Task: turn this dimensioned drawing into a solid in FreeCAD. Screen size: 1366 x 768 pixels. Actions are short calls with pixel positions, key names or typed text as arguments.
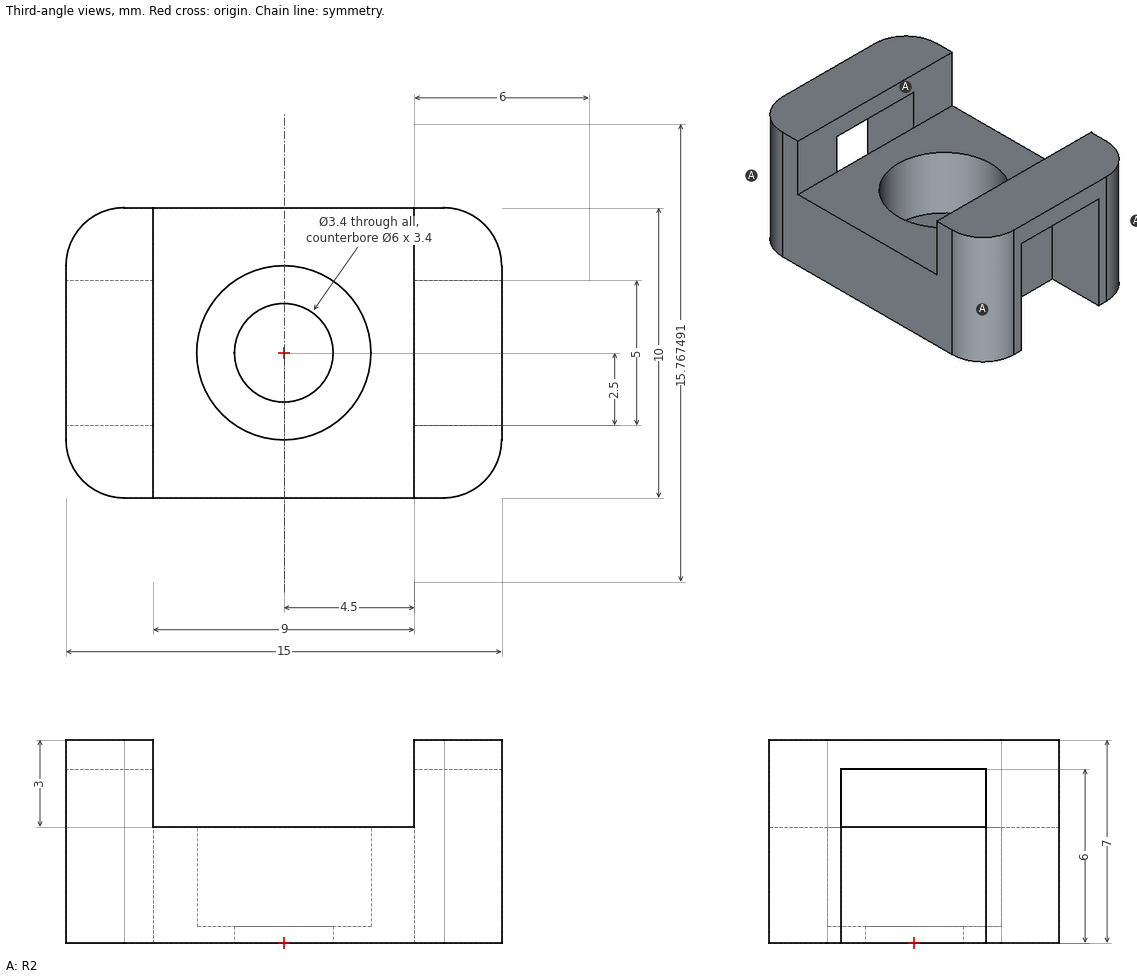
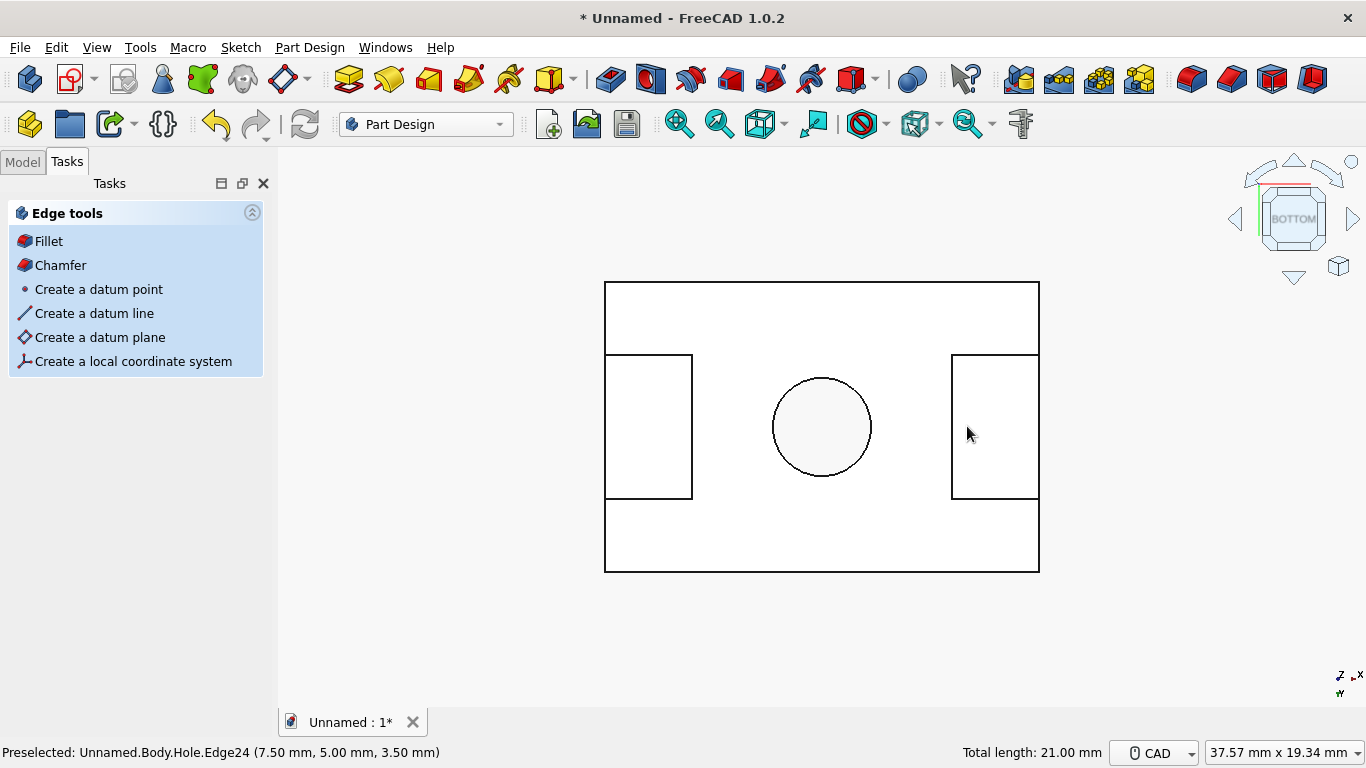
key(4)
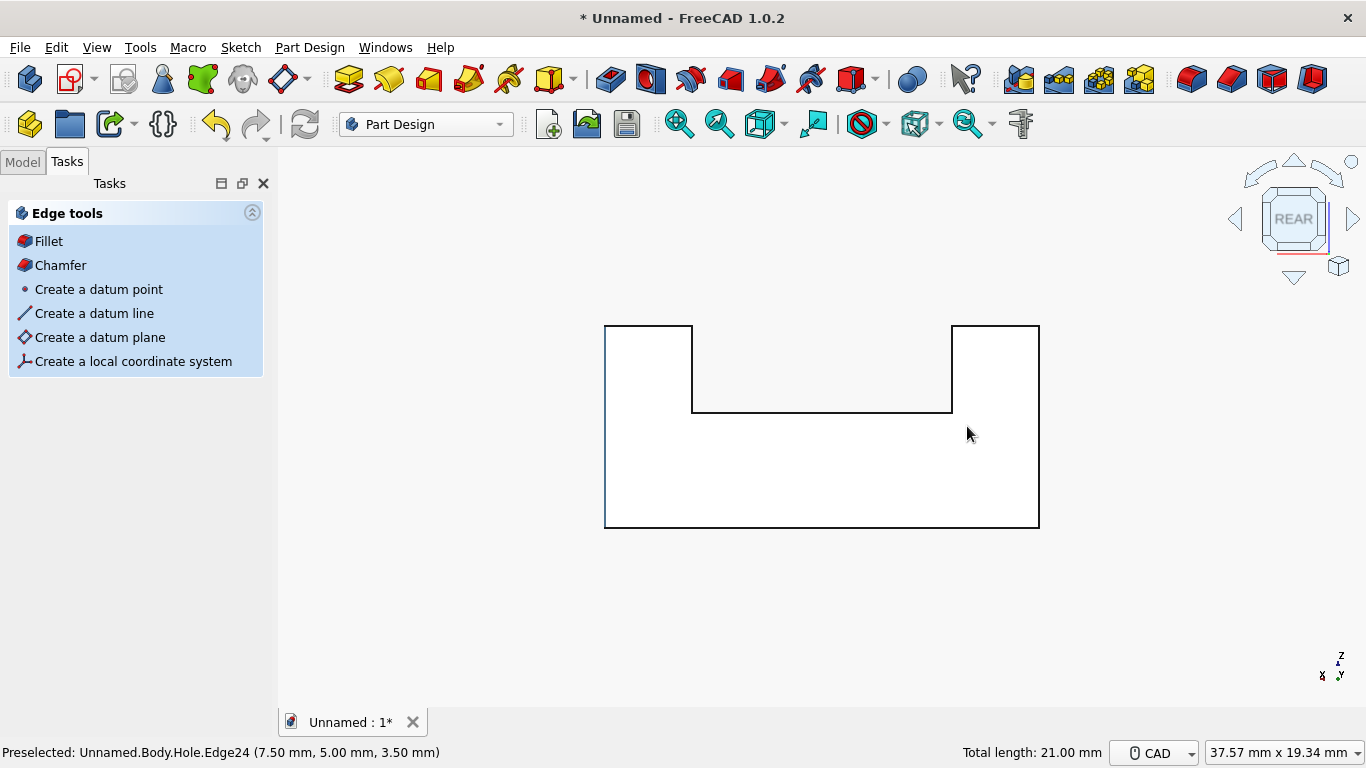
click(680, 124)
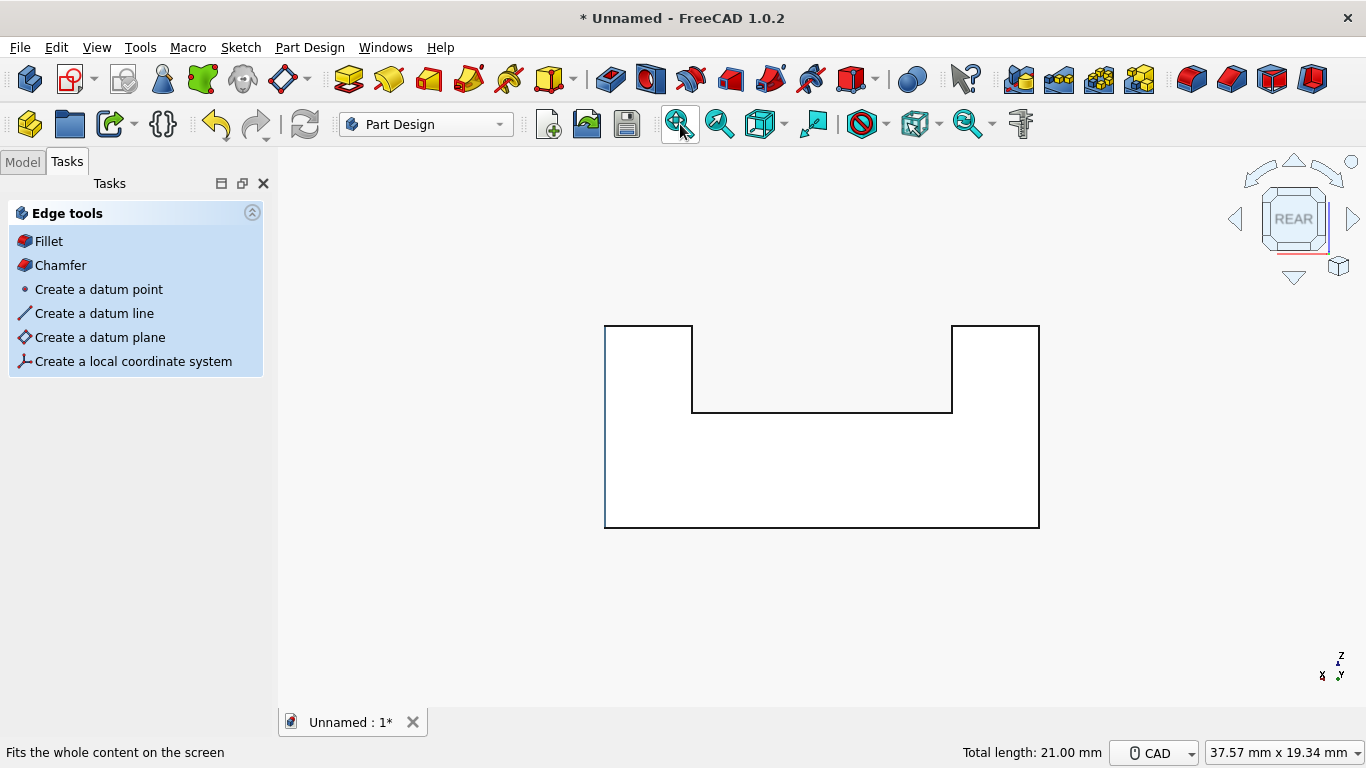
click(1039, 426, ctrl)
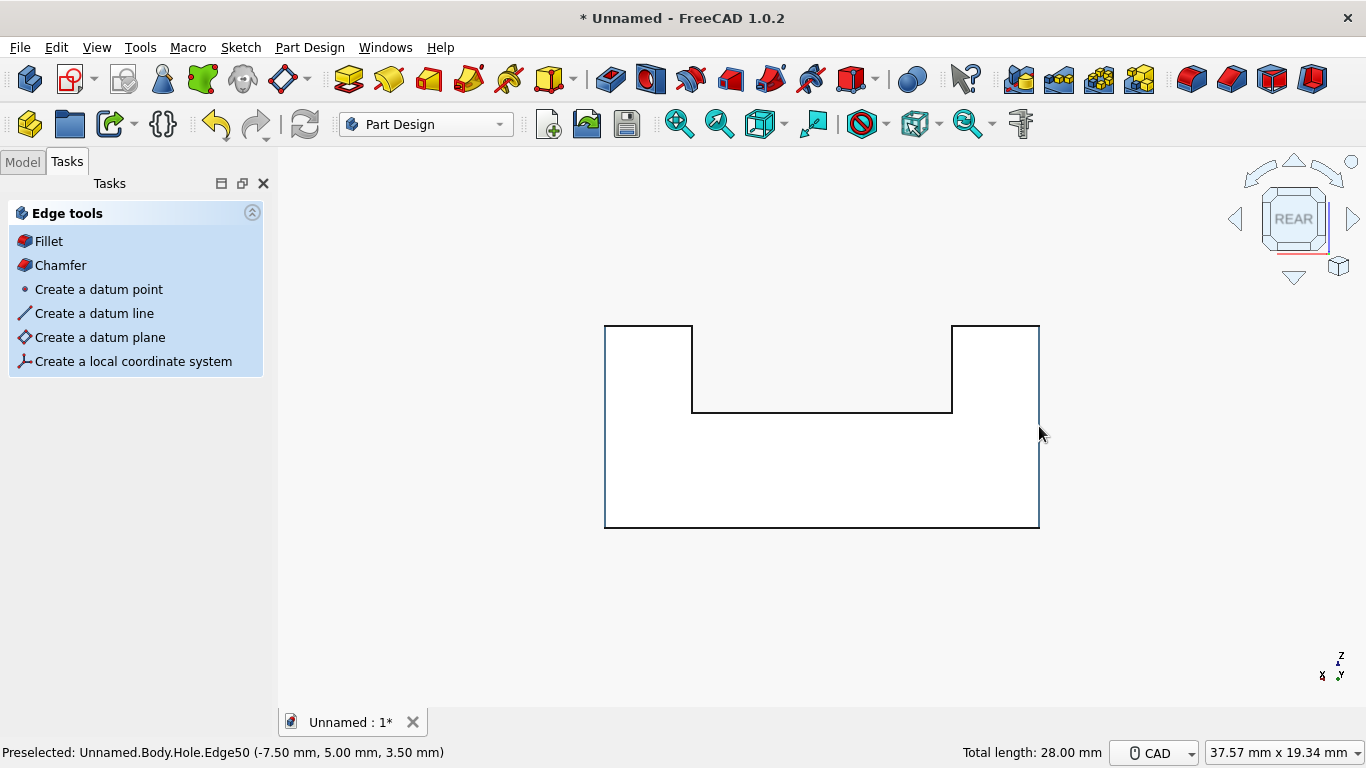
click(1192, 80)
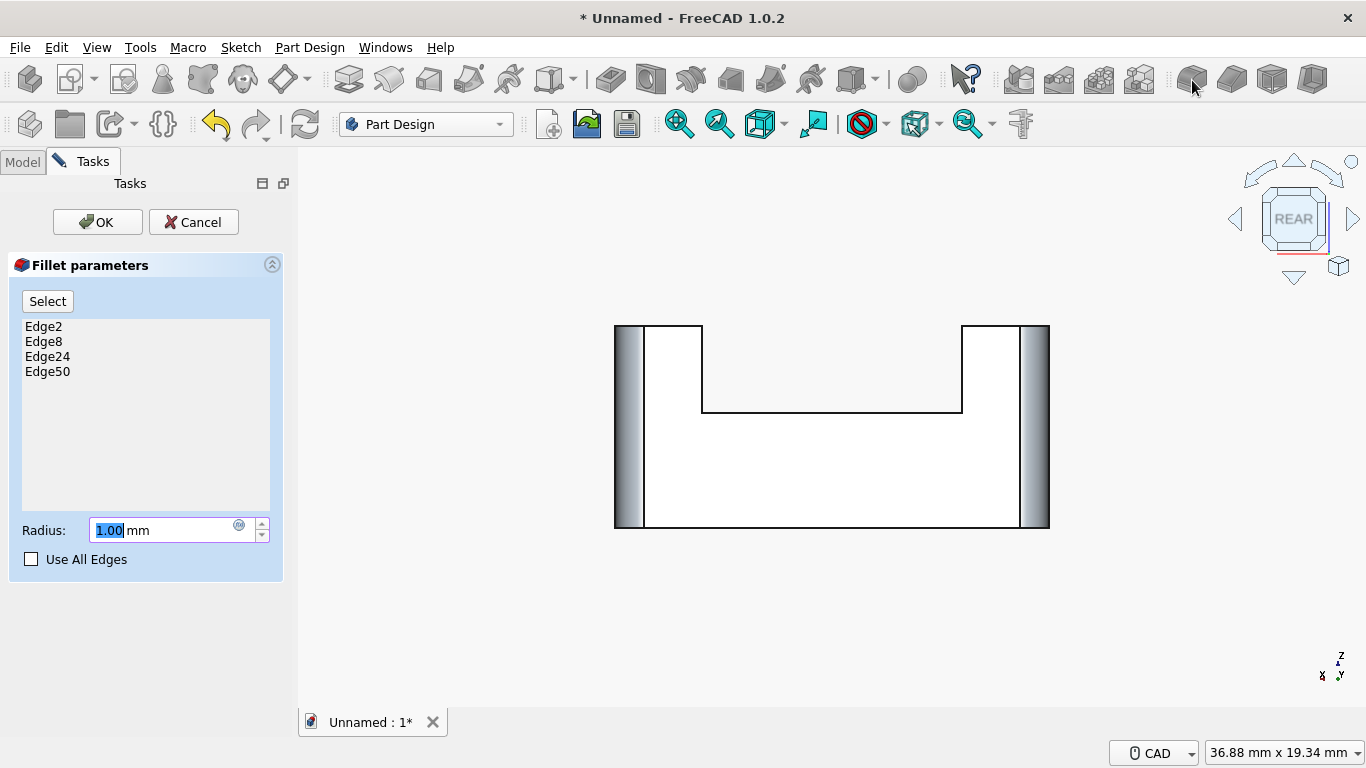
text(2)
key(Tab)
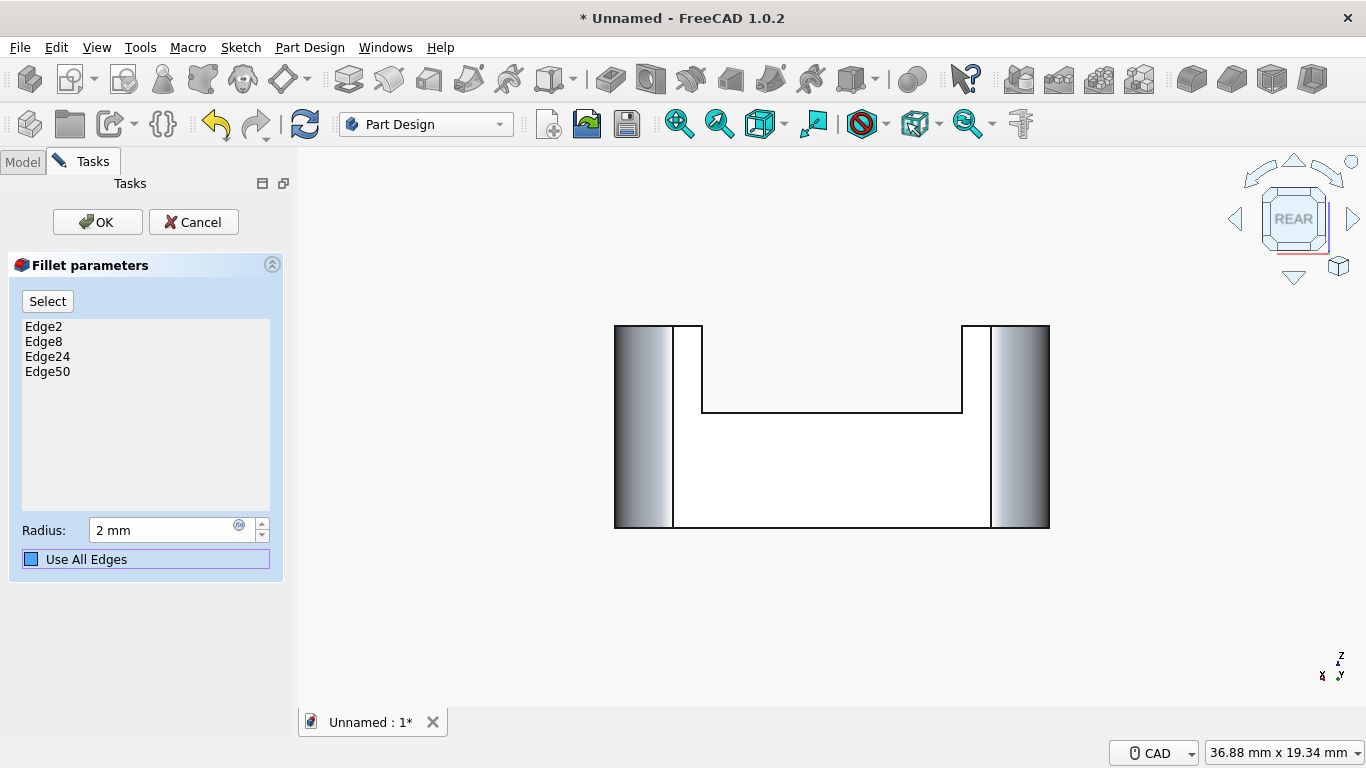
click(98, 222)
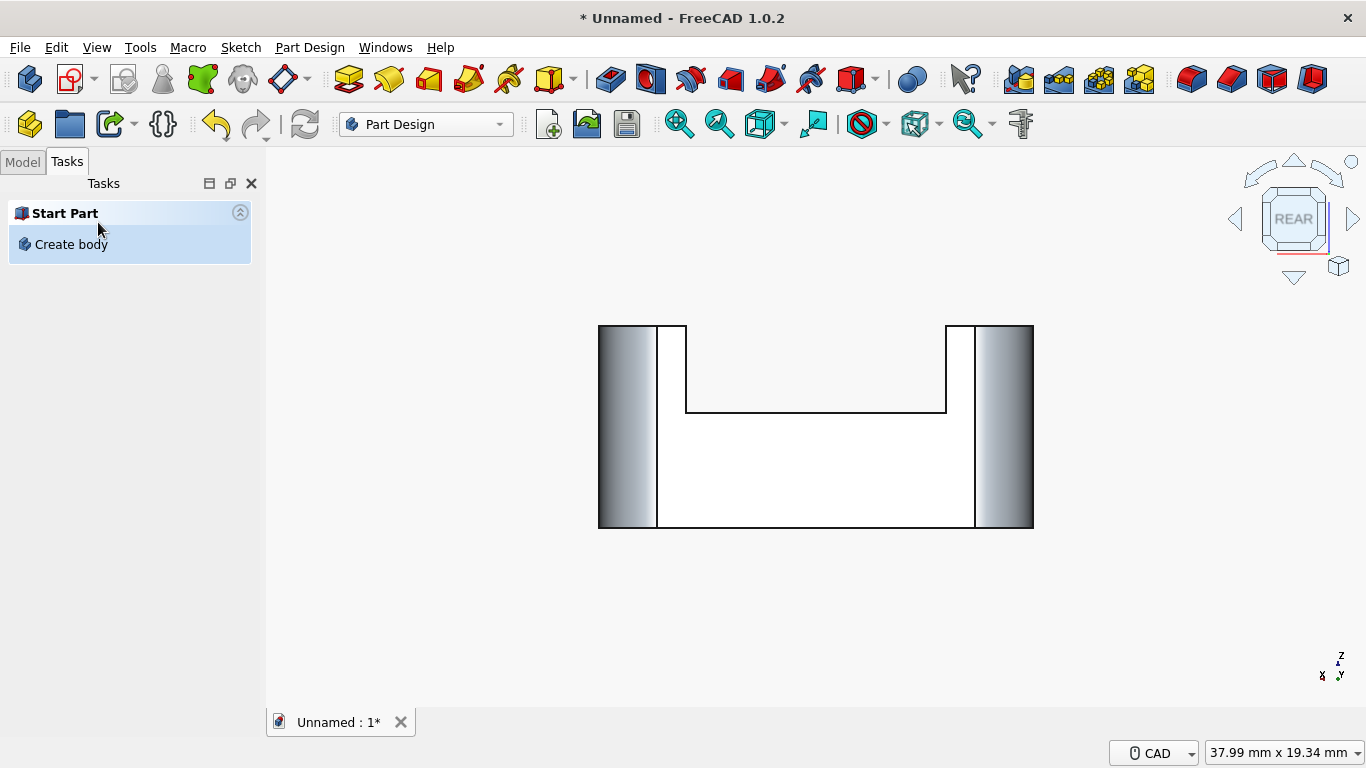
key(0)